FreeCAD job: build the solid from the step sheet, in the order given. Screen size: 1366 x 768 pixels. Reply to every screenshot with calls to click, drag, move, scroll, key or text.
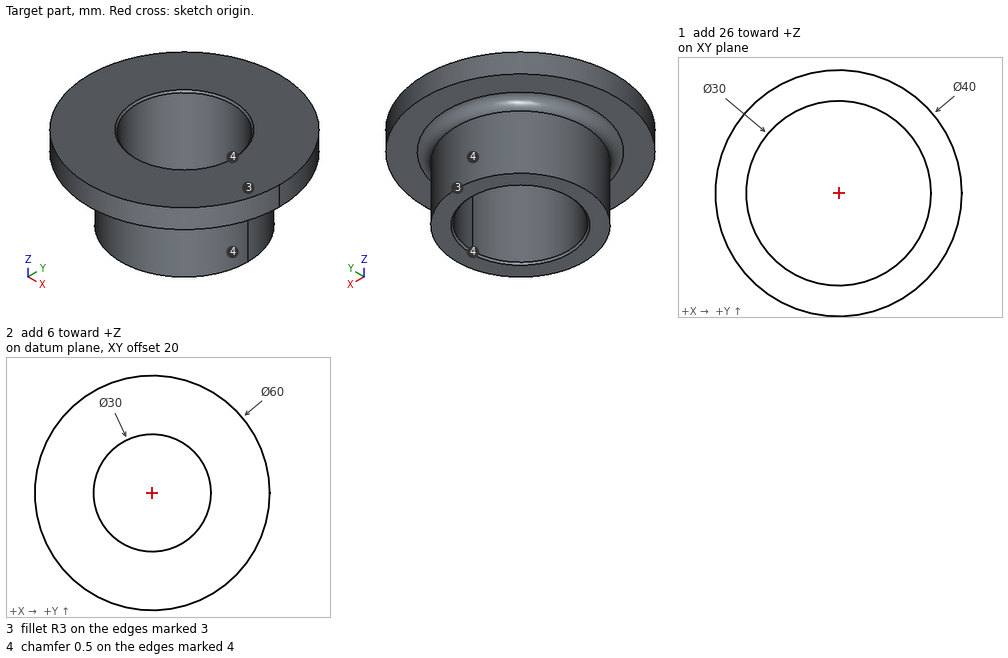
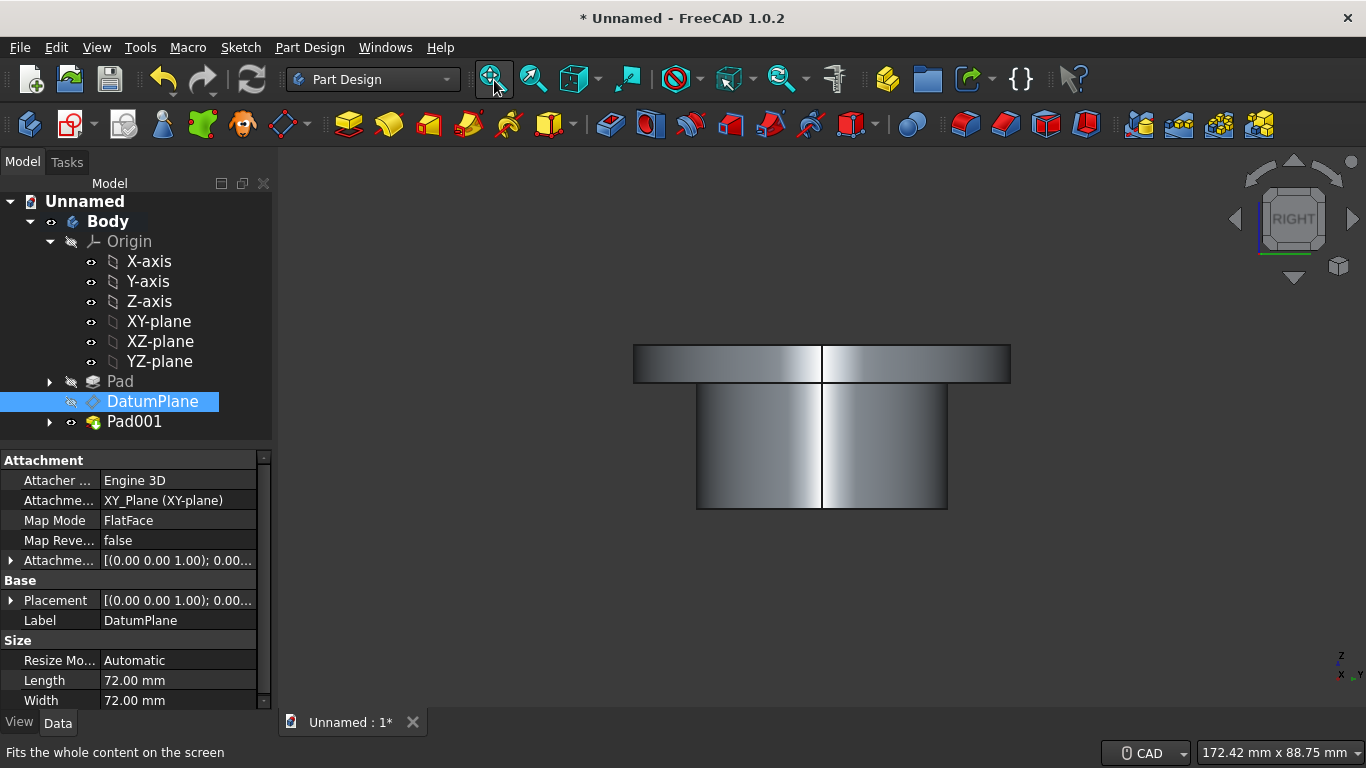
click(494, 80)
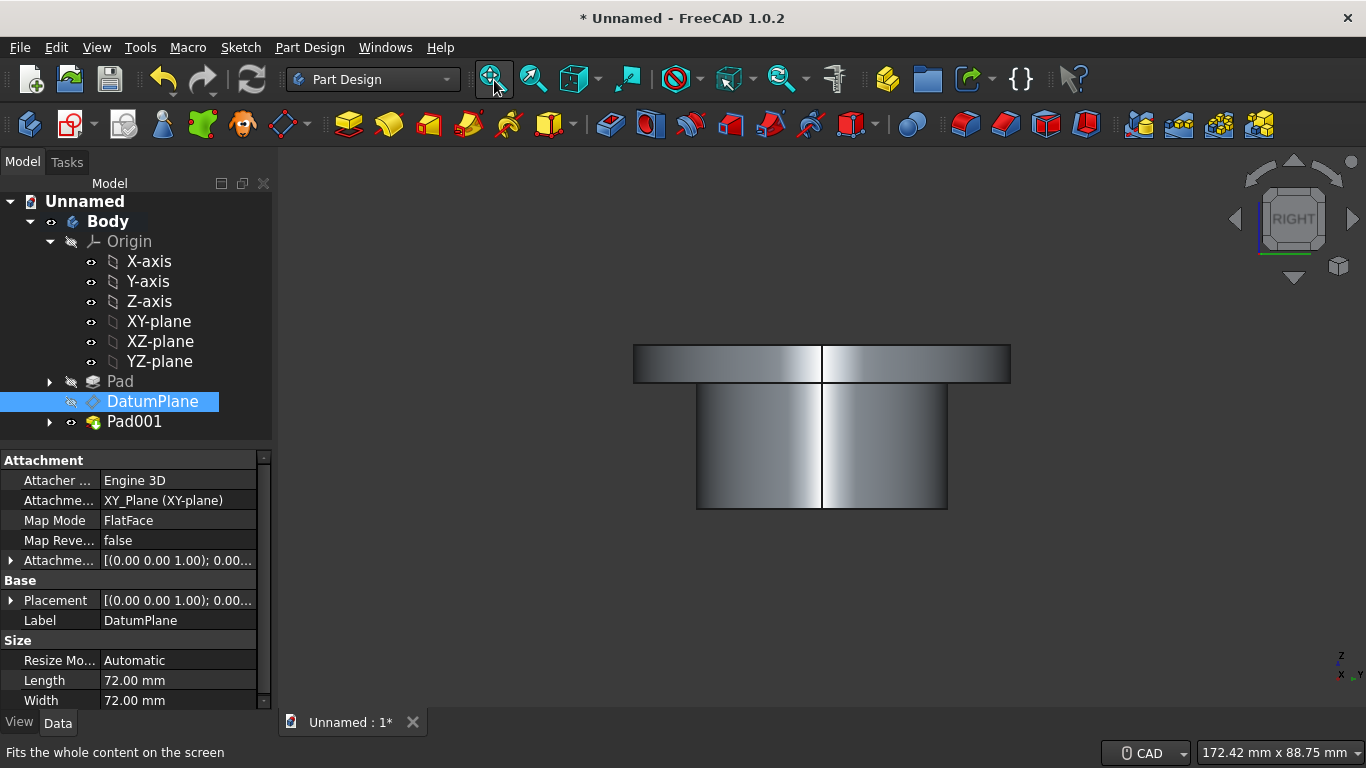
key(5)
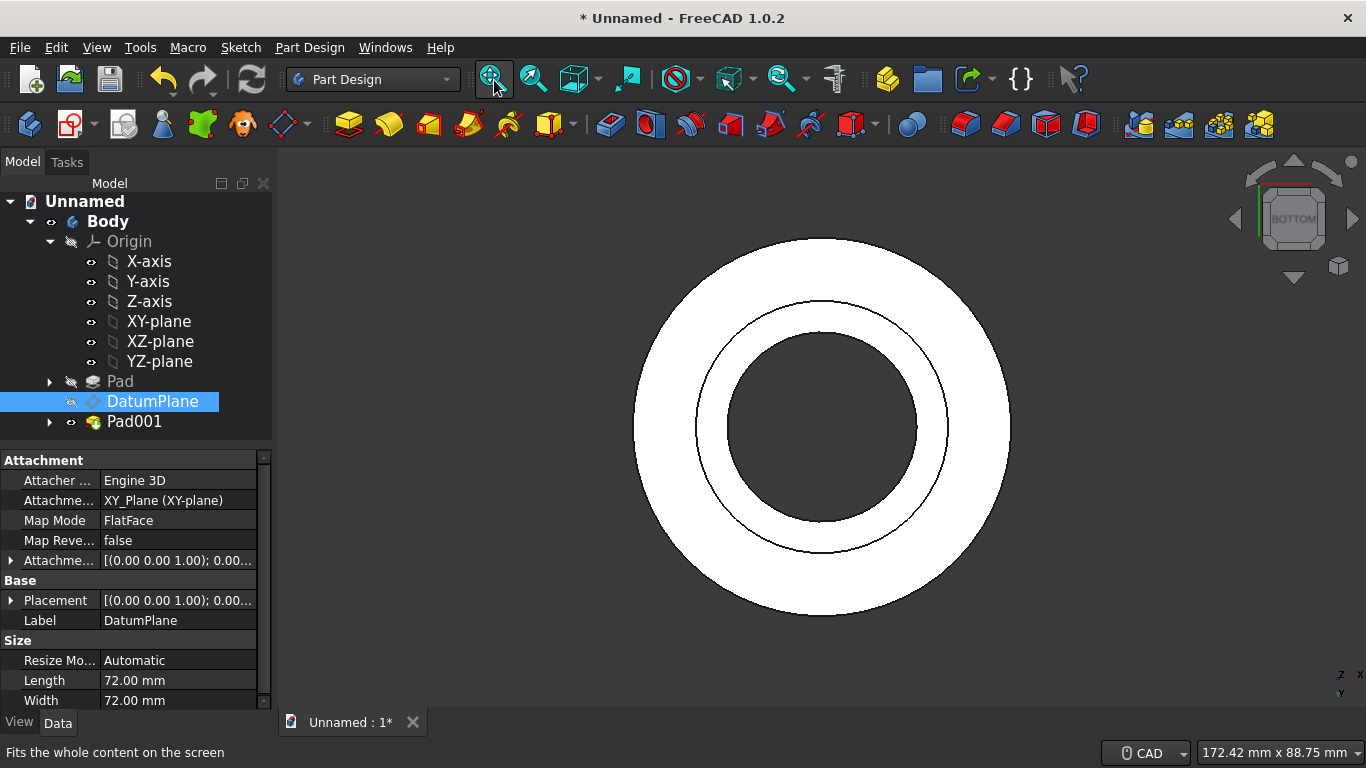
key(4)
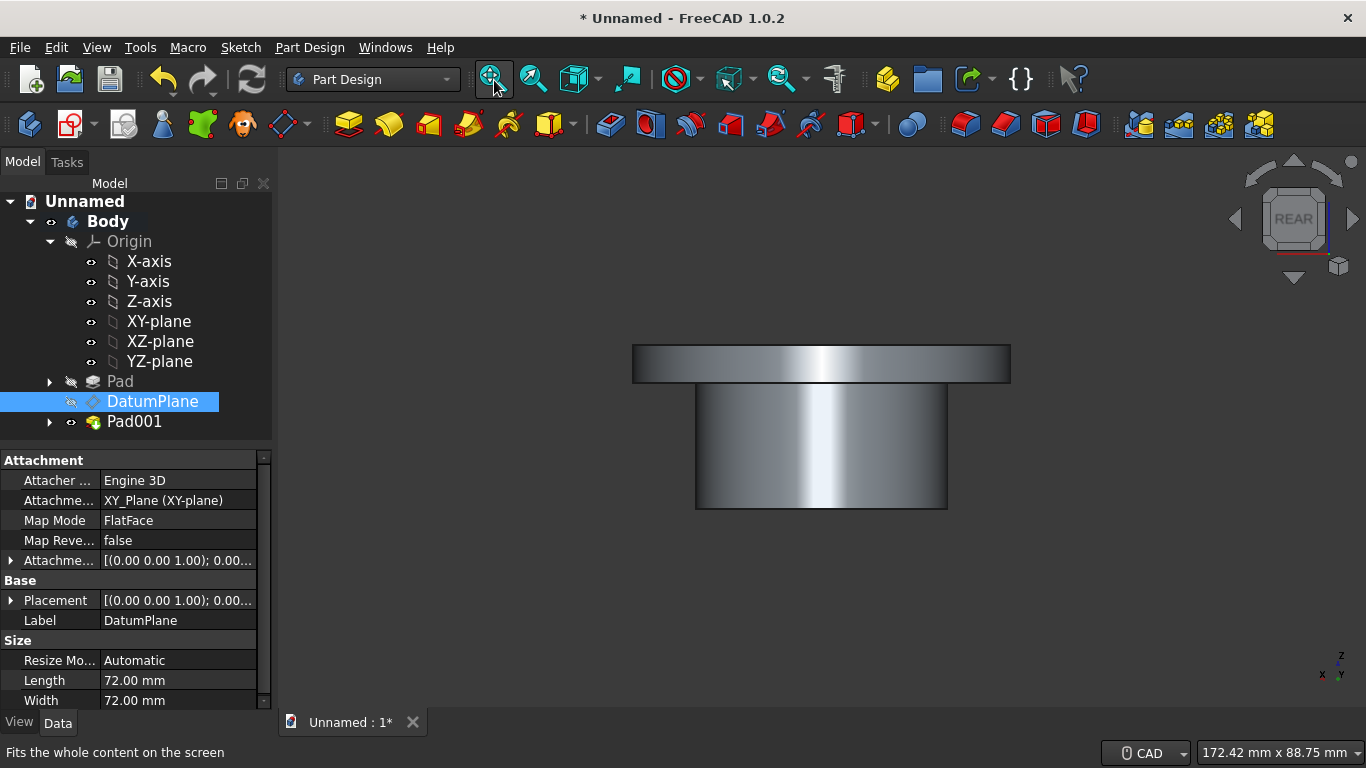
click(494, 80)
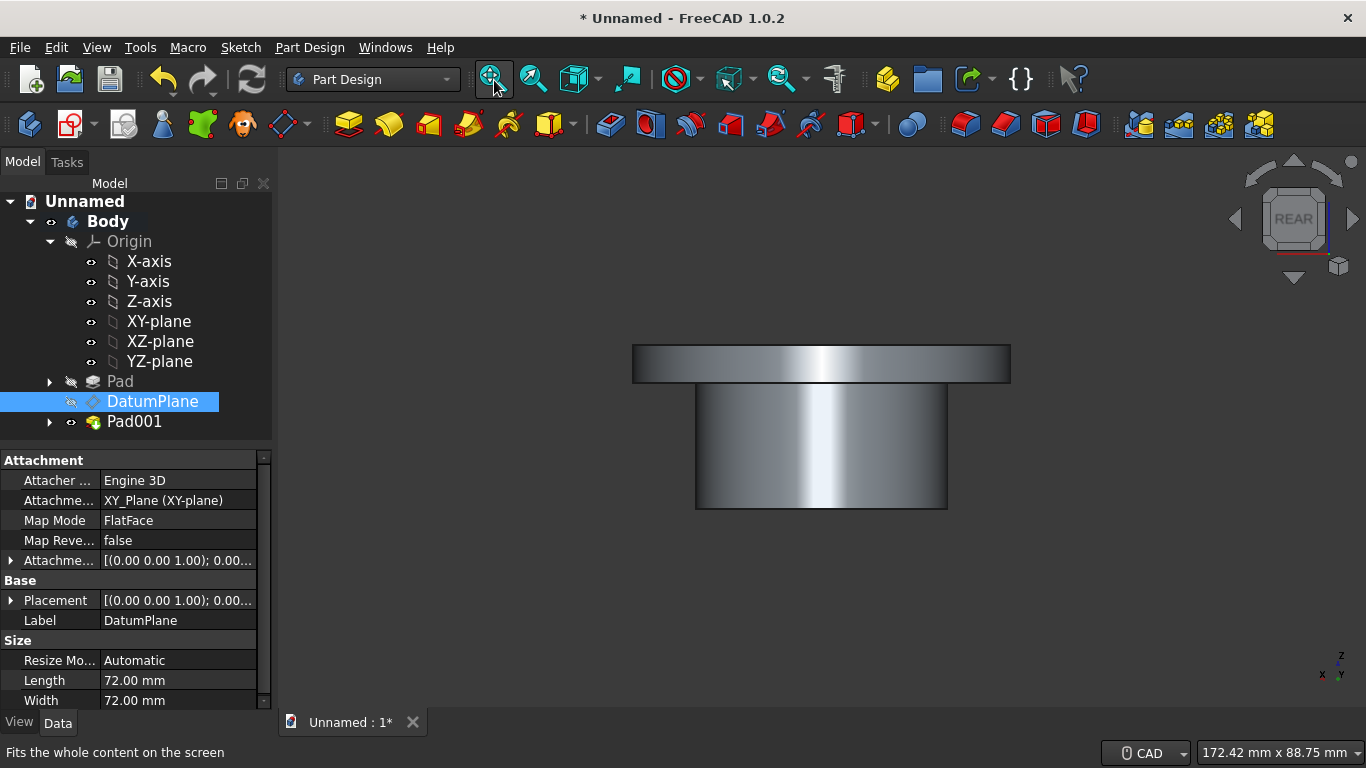
key(6)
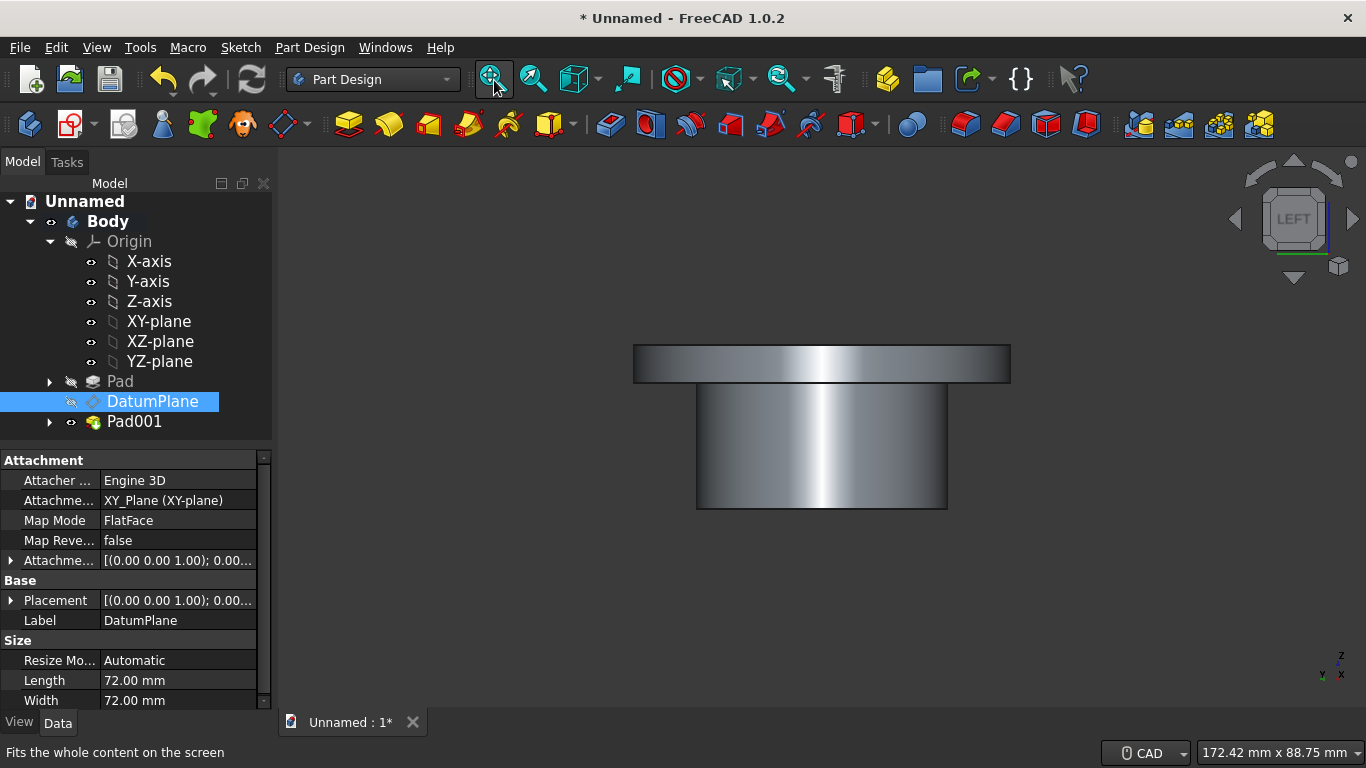
key(v)
key(f)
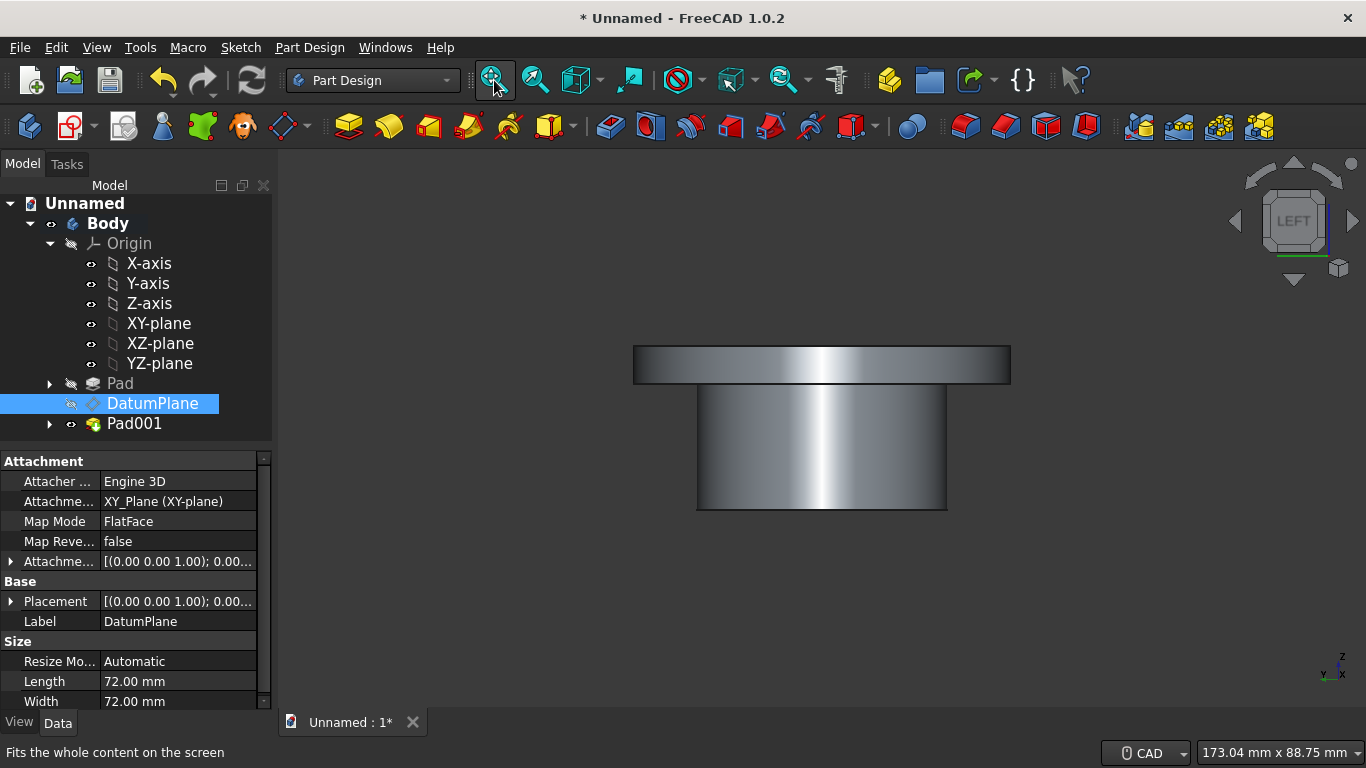
key(v)
key(3)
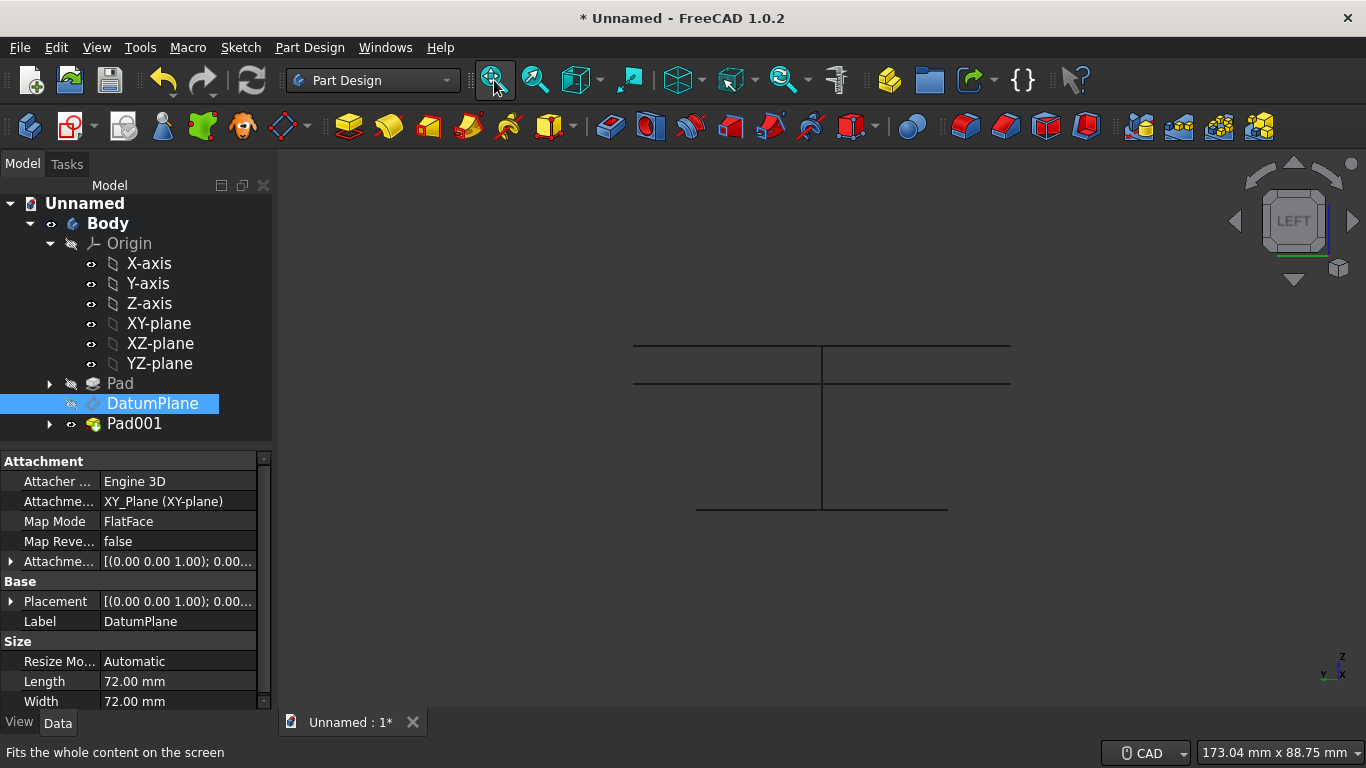
key(0)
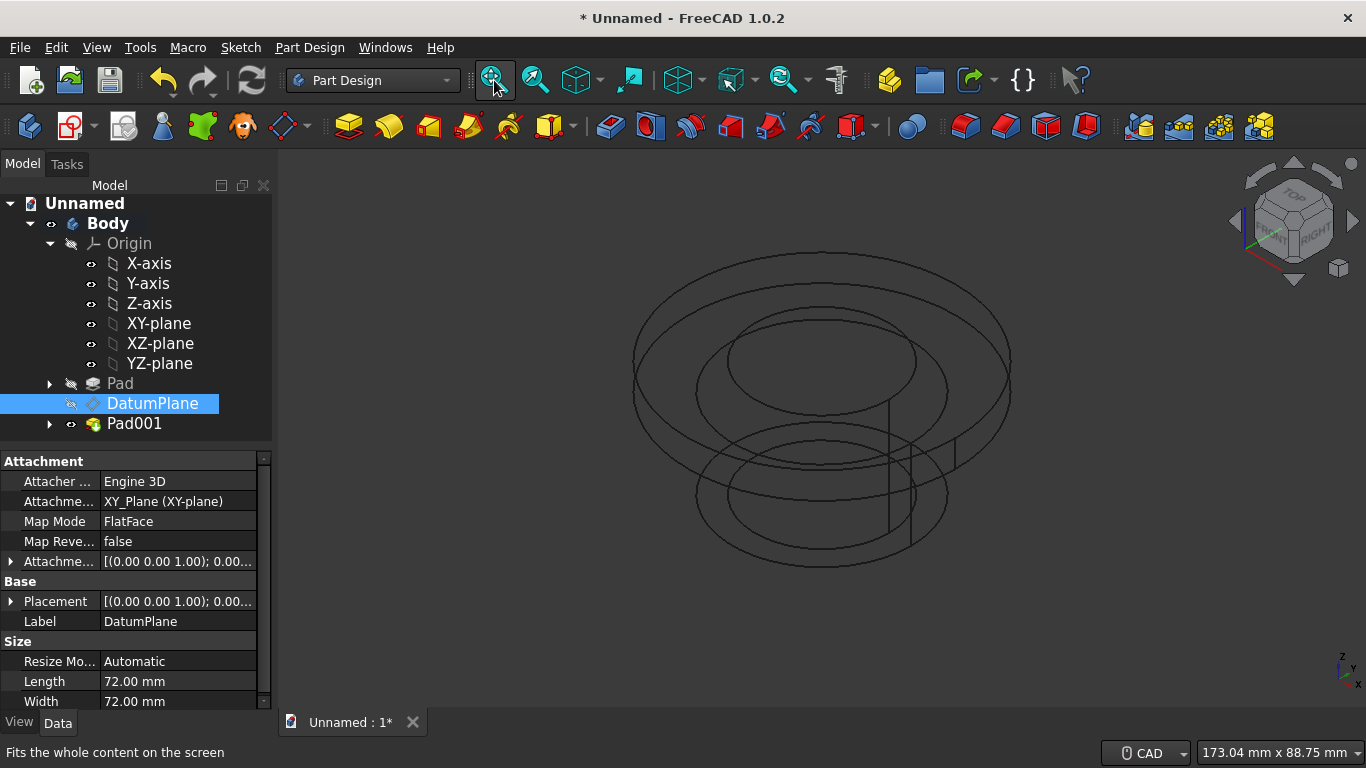
click(698, 380)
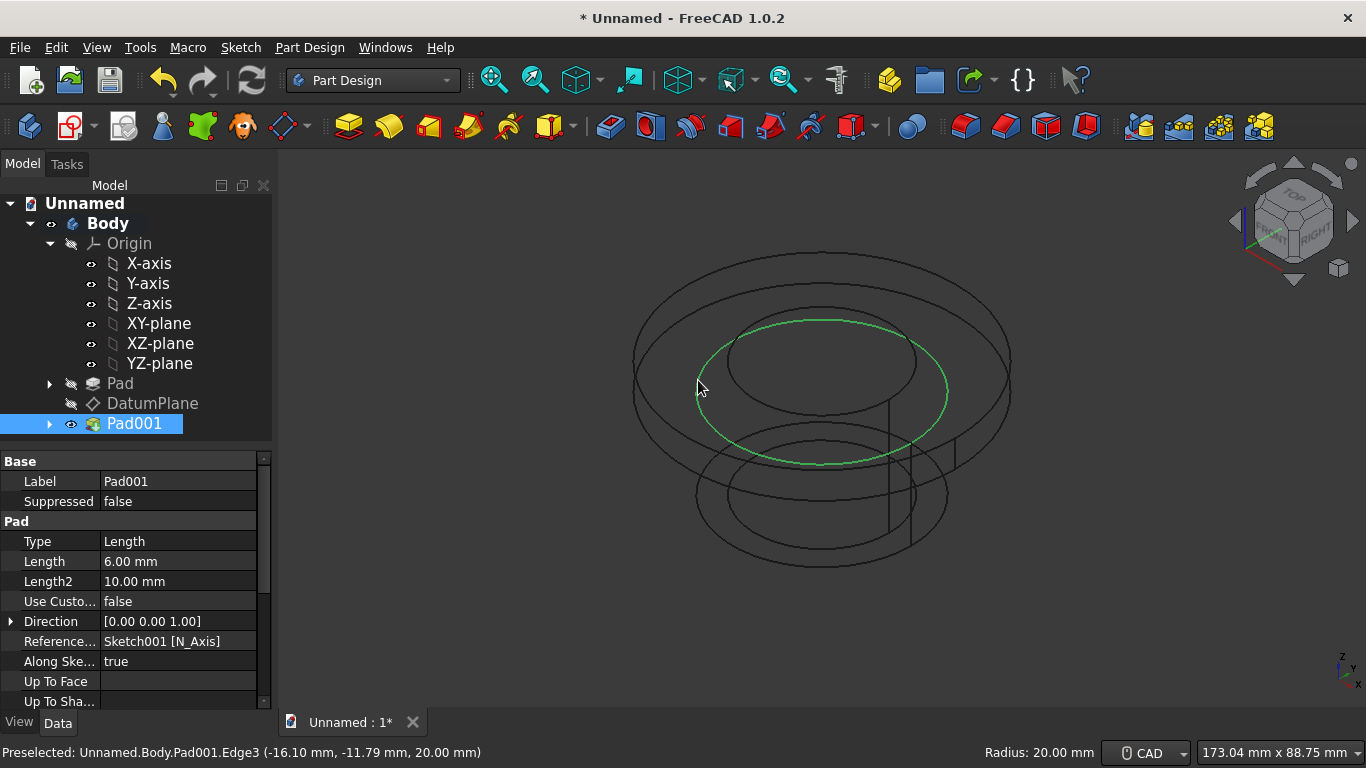
key(v)
key(1)